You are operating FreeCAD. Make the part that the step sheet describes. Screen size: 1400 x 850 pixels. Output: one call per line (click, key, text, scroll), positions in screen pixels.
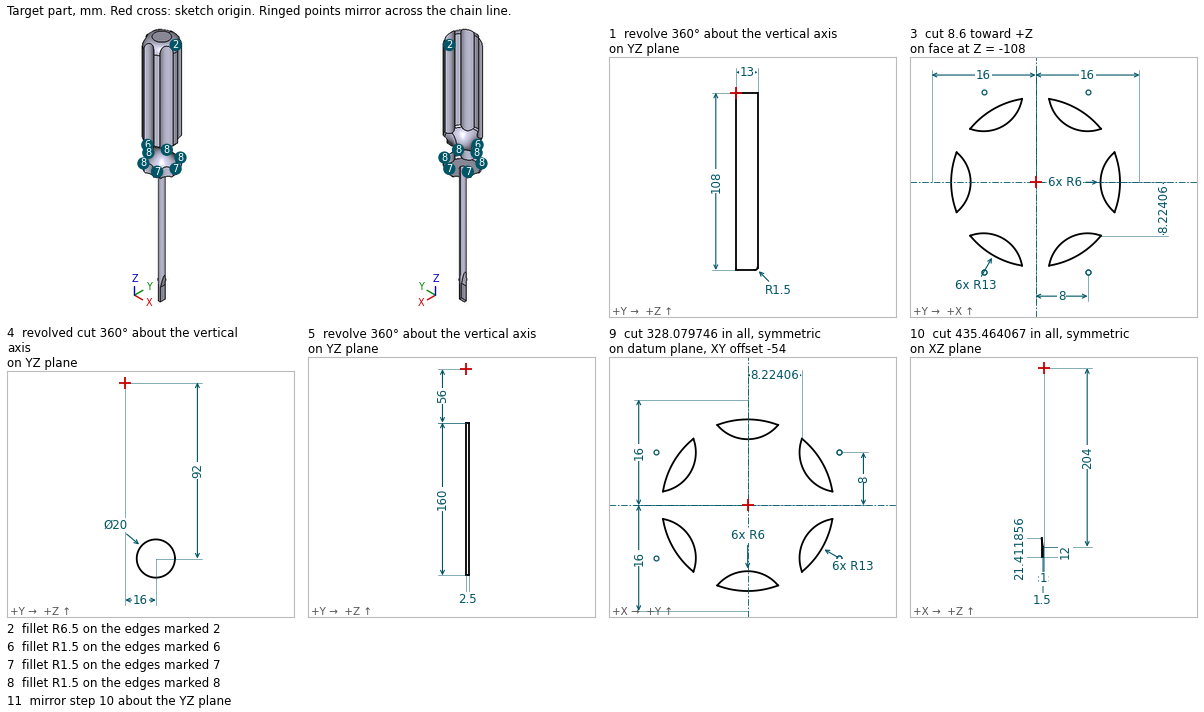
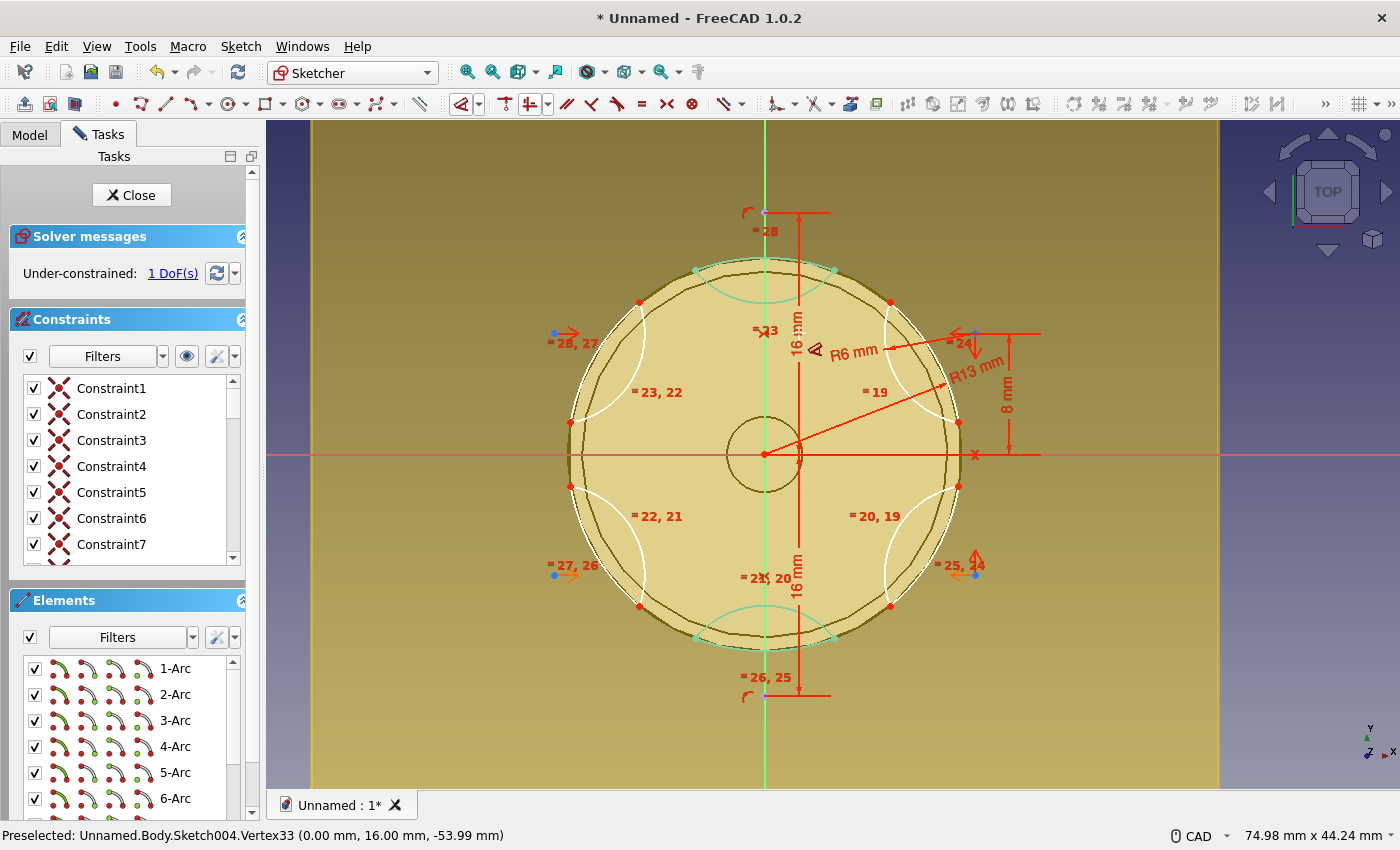
click(890, 303)
click(856, 269)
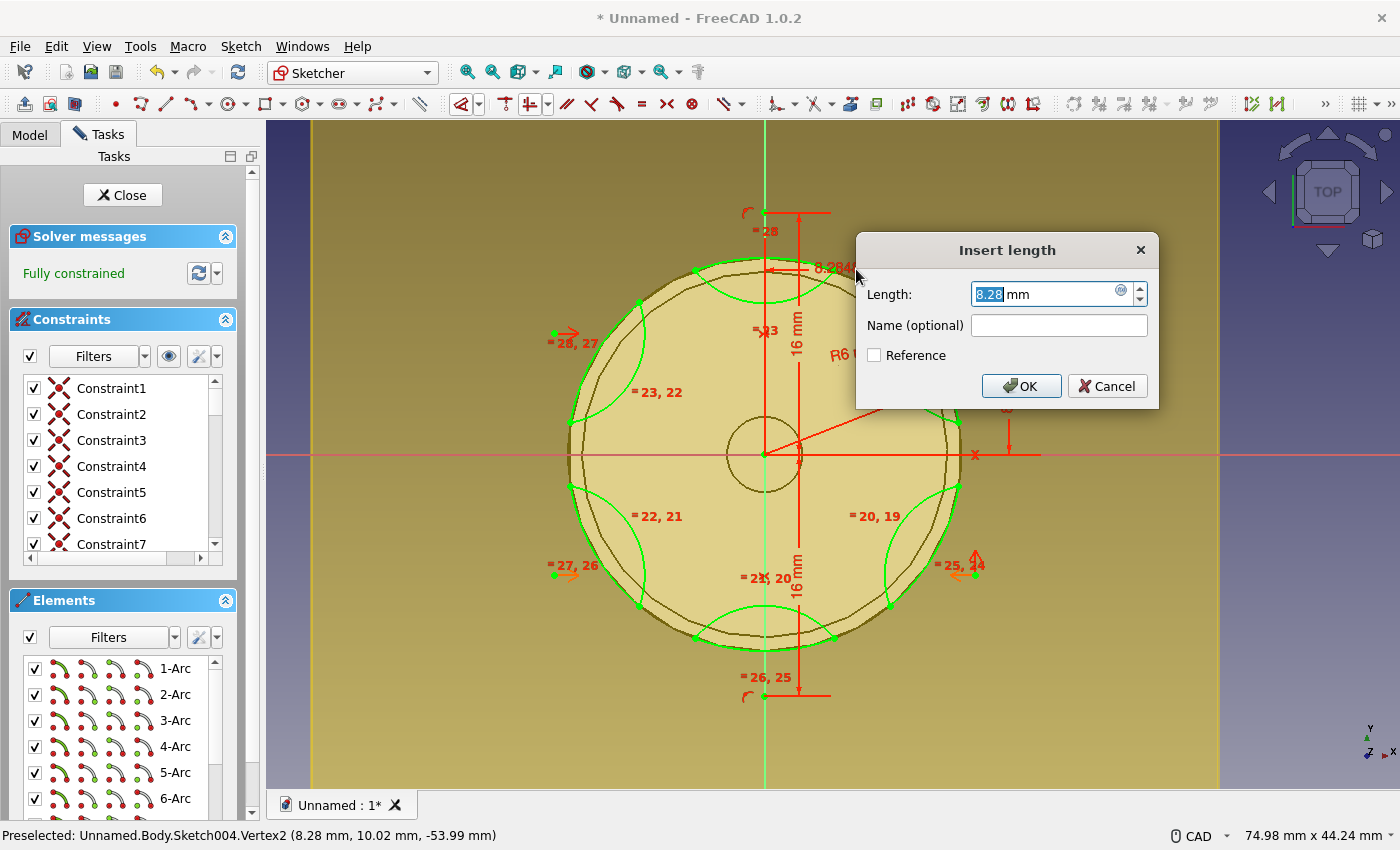
text(8.22406)
key(Return)
key(Escape)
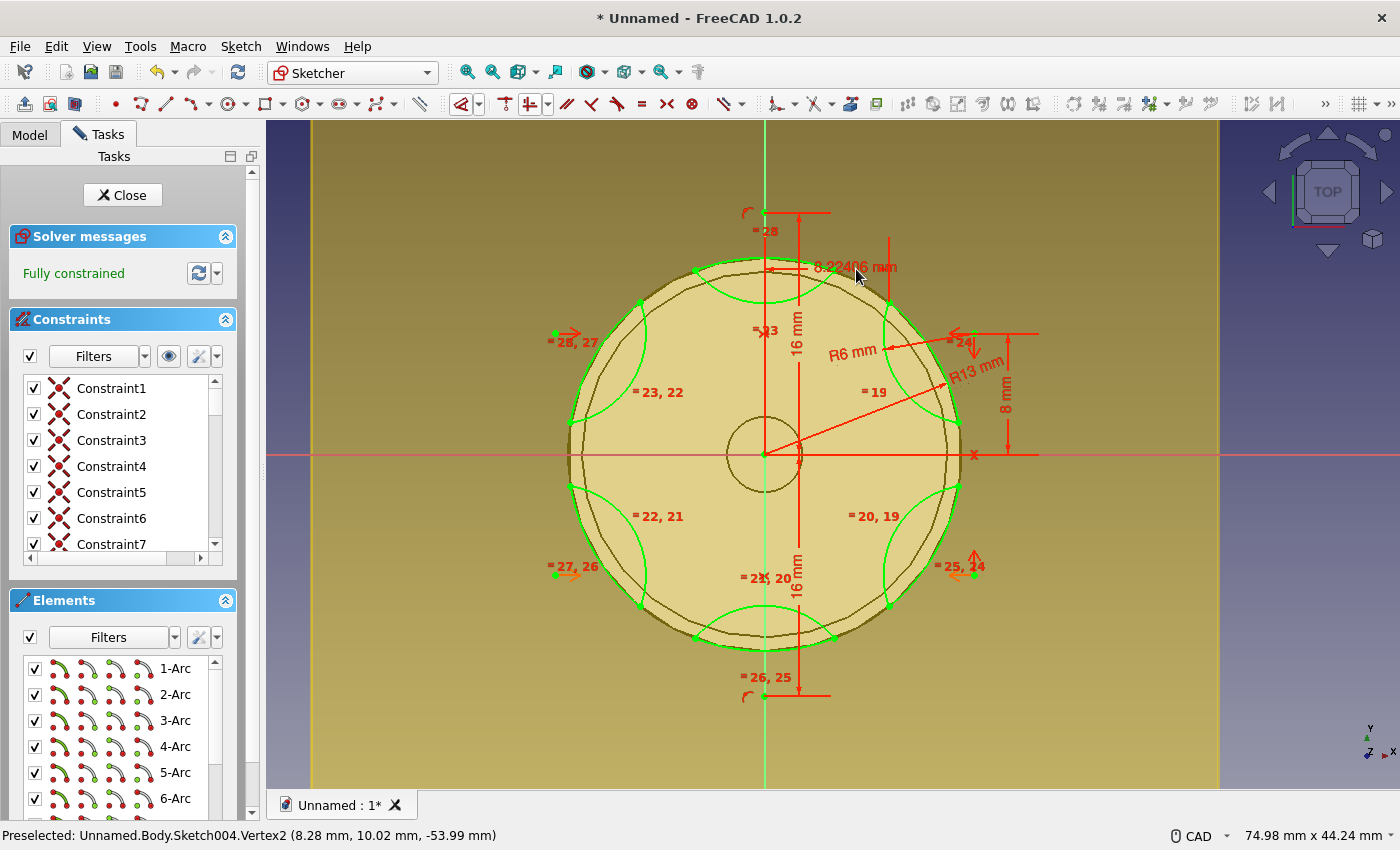
click(123, 195)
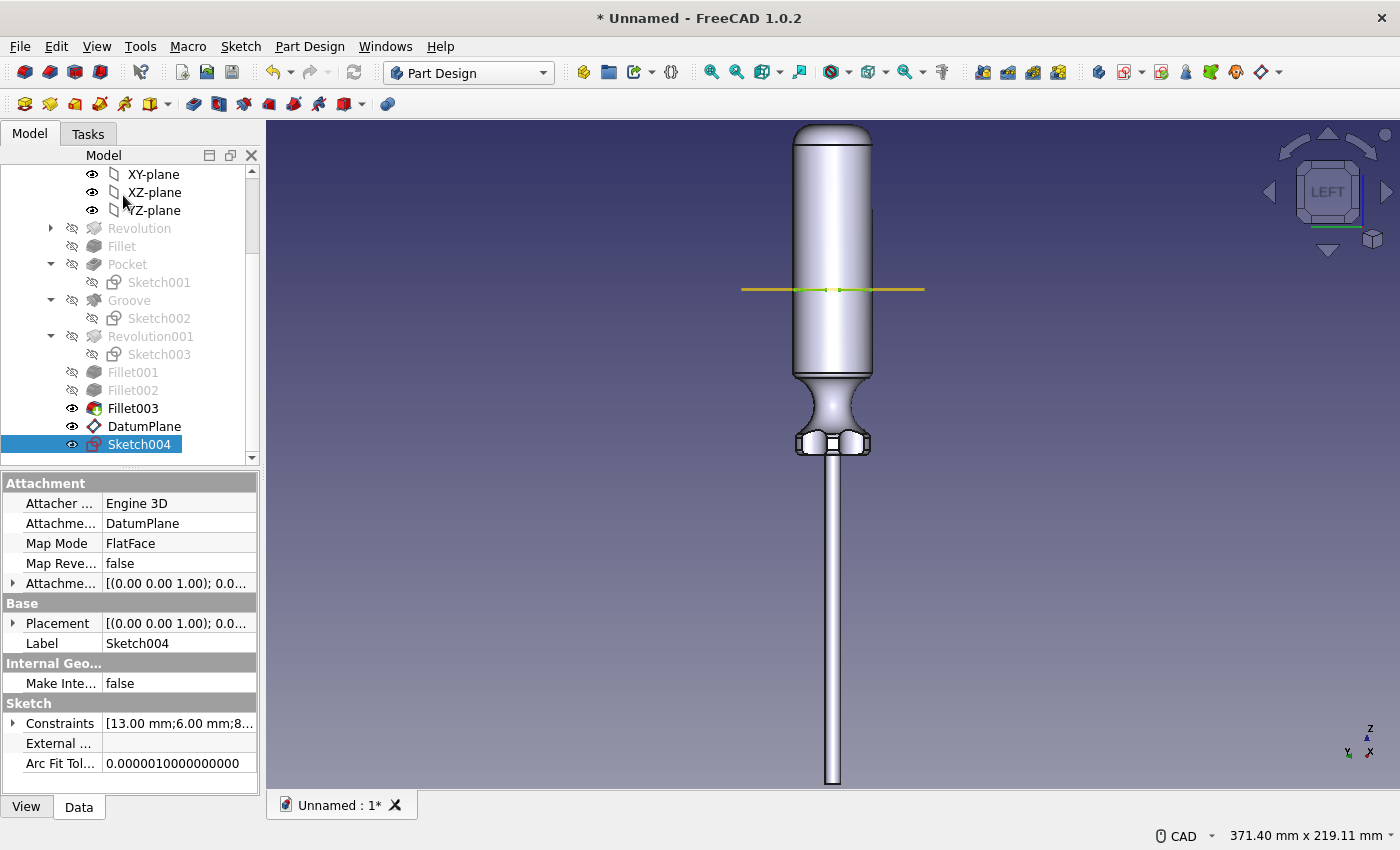
click(194, 104)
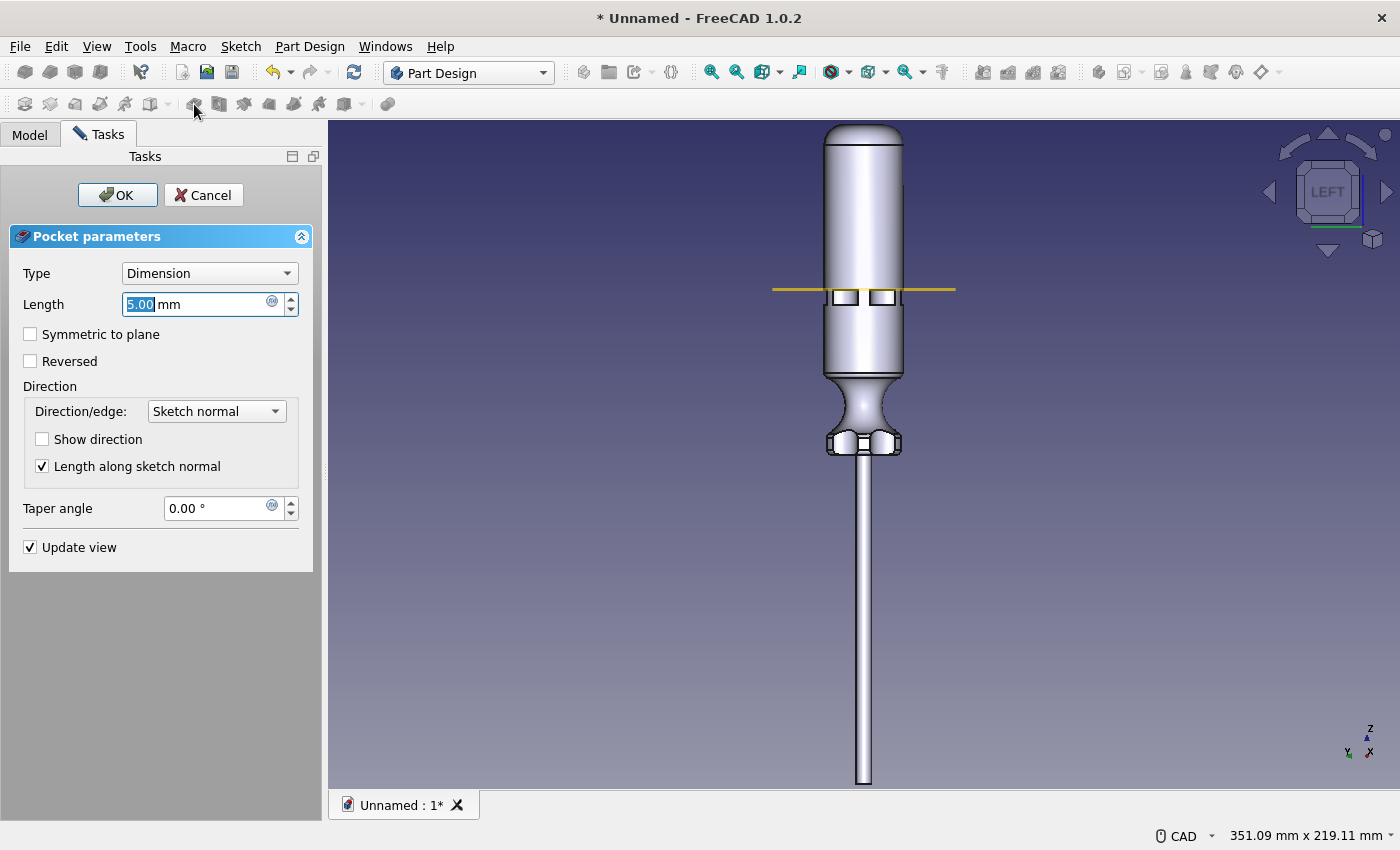
text(328.079746)
key(Tab)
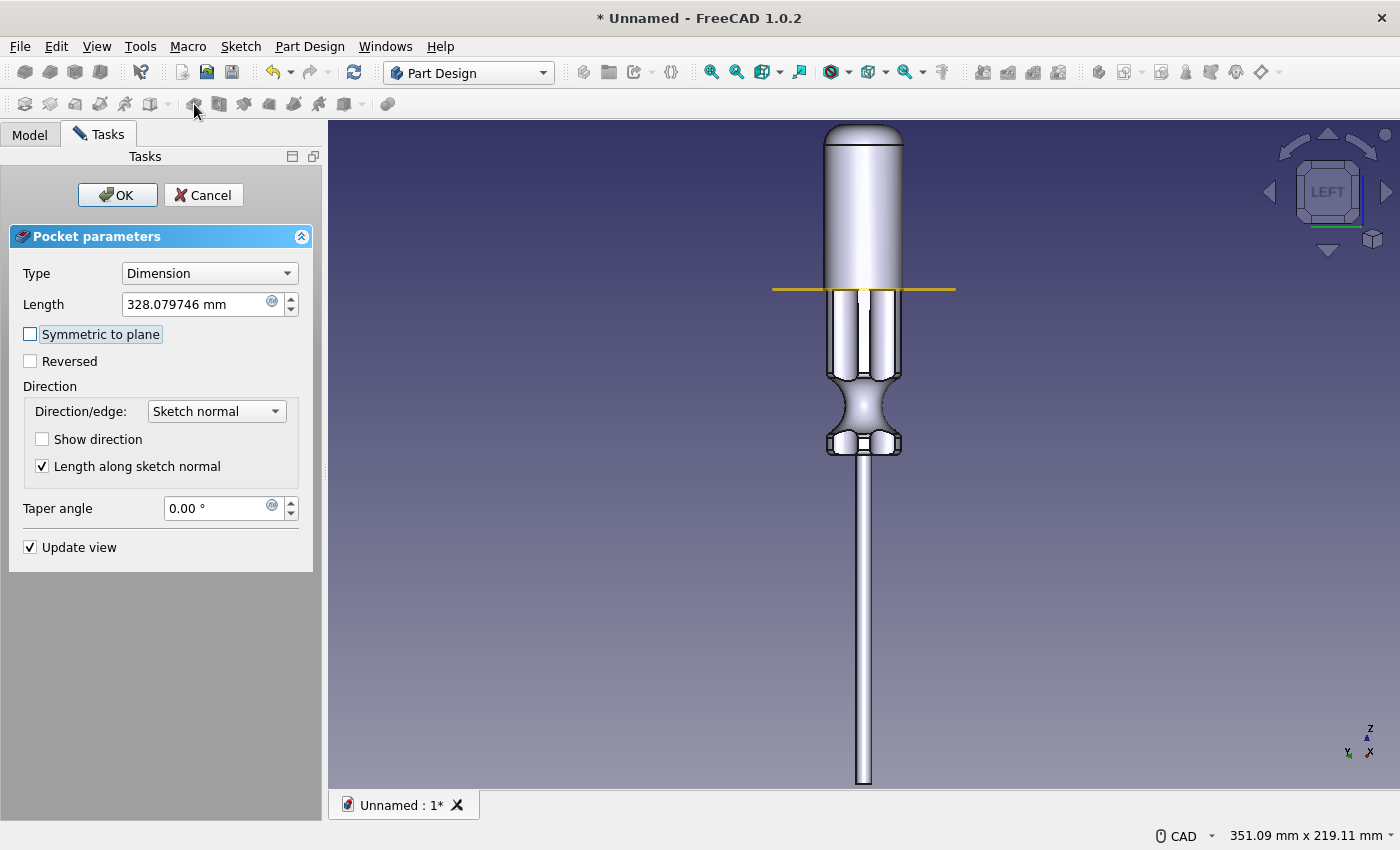
click(31, 334)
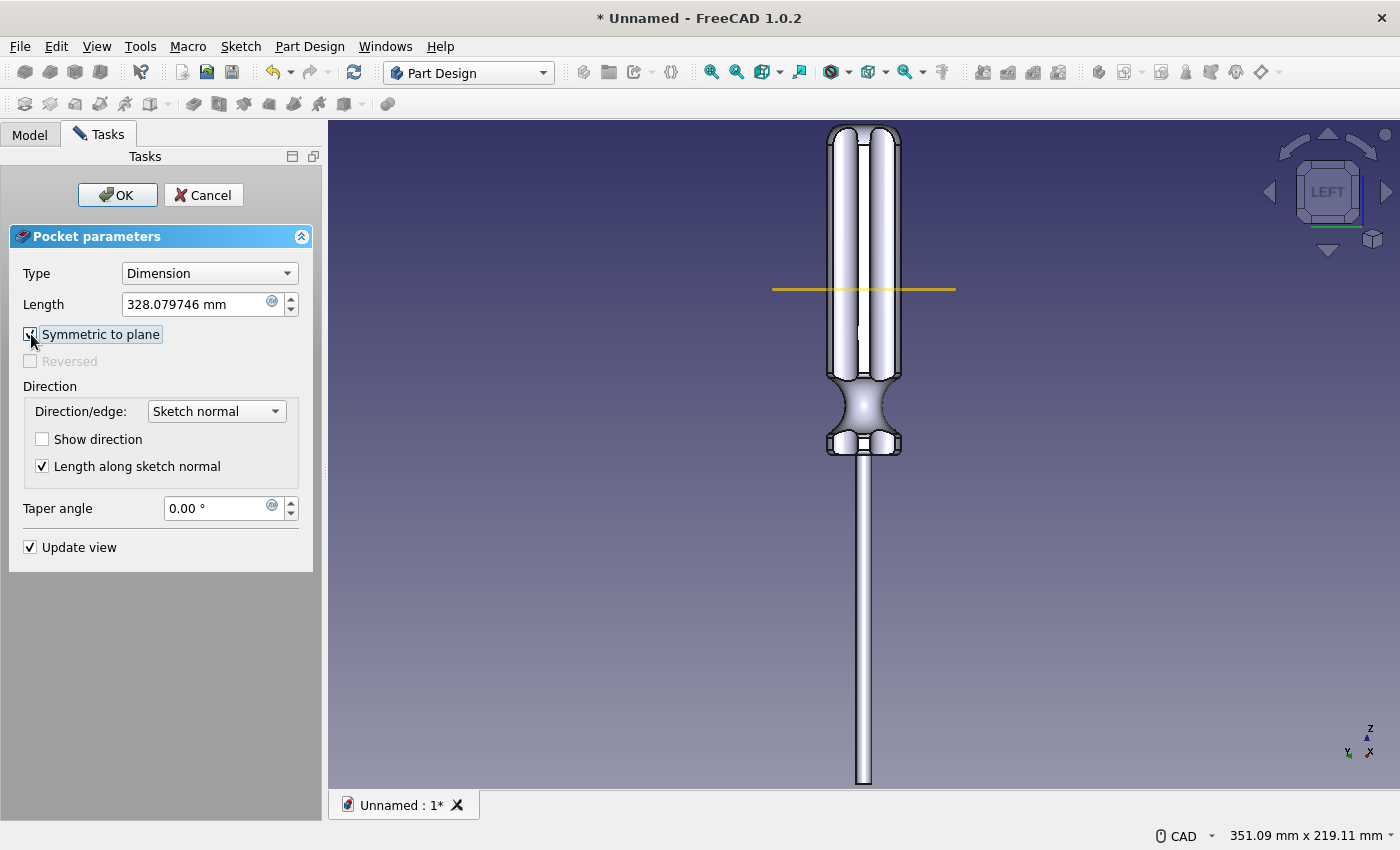
click(118, 195)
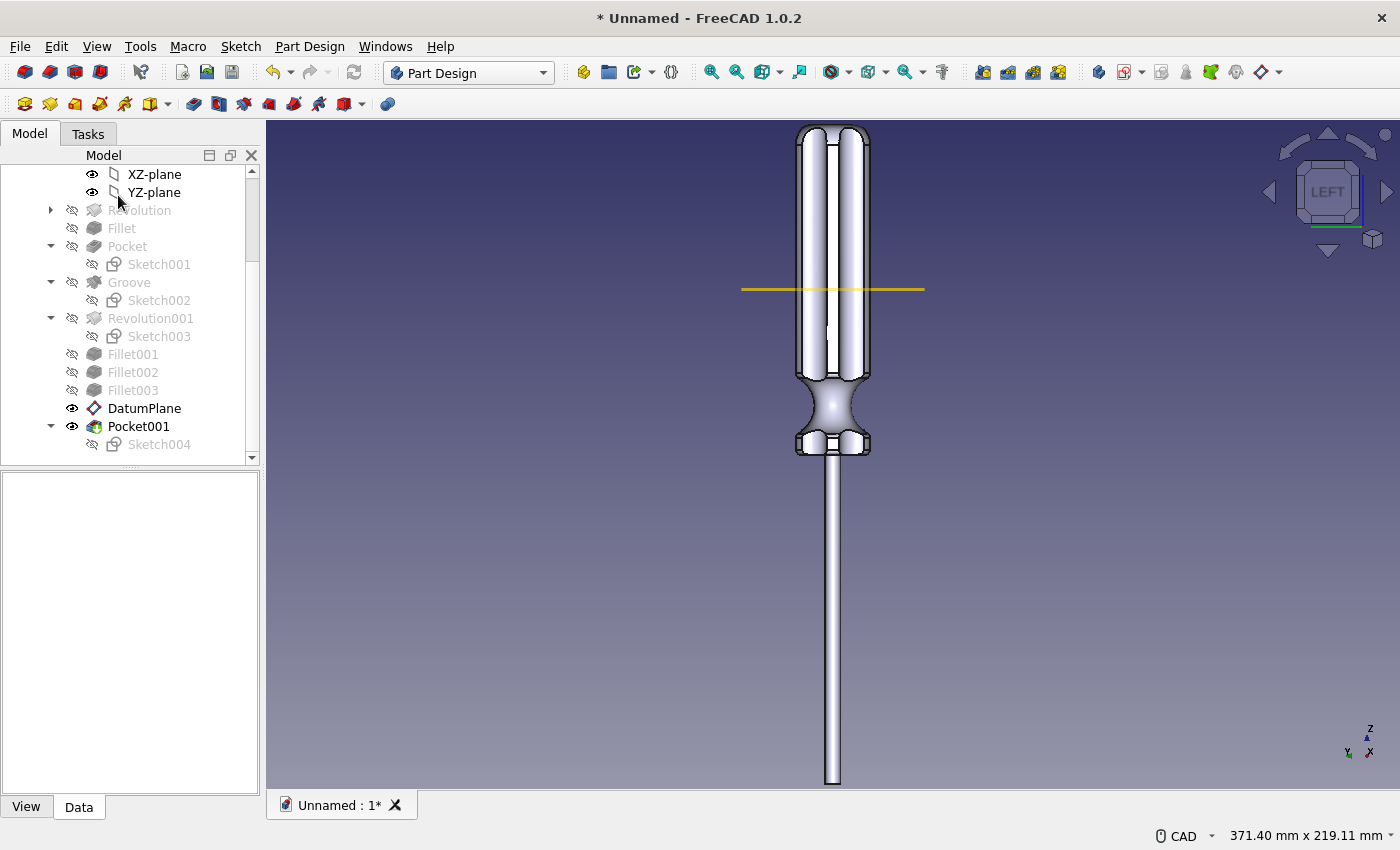
click(117, 408)
key(space)